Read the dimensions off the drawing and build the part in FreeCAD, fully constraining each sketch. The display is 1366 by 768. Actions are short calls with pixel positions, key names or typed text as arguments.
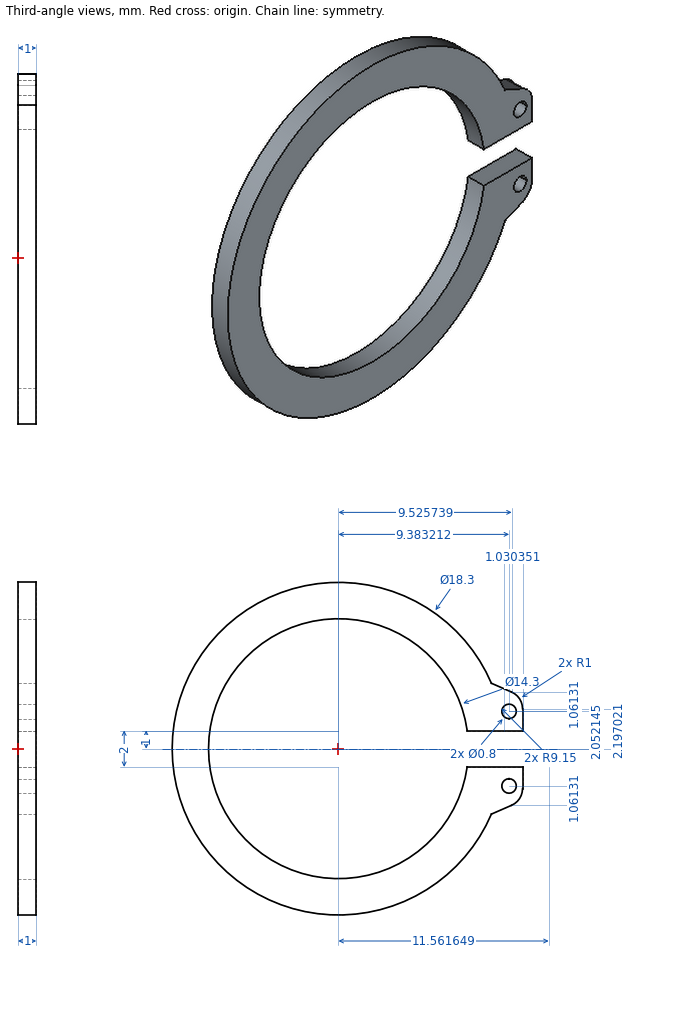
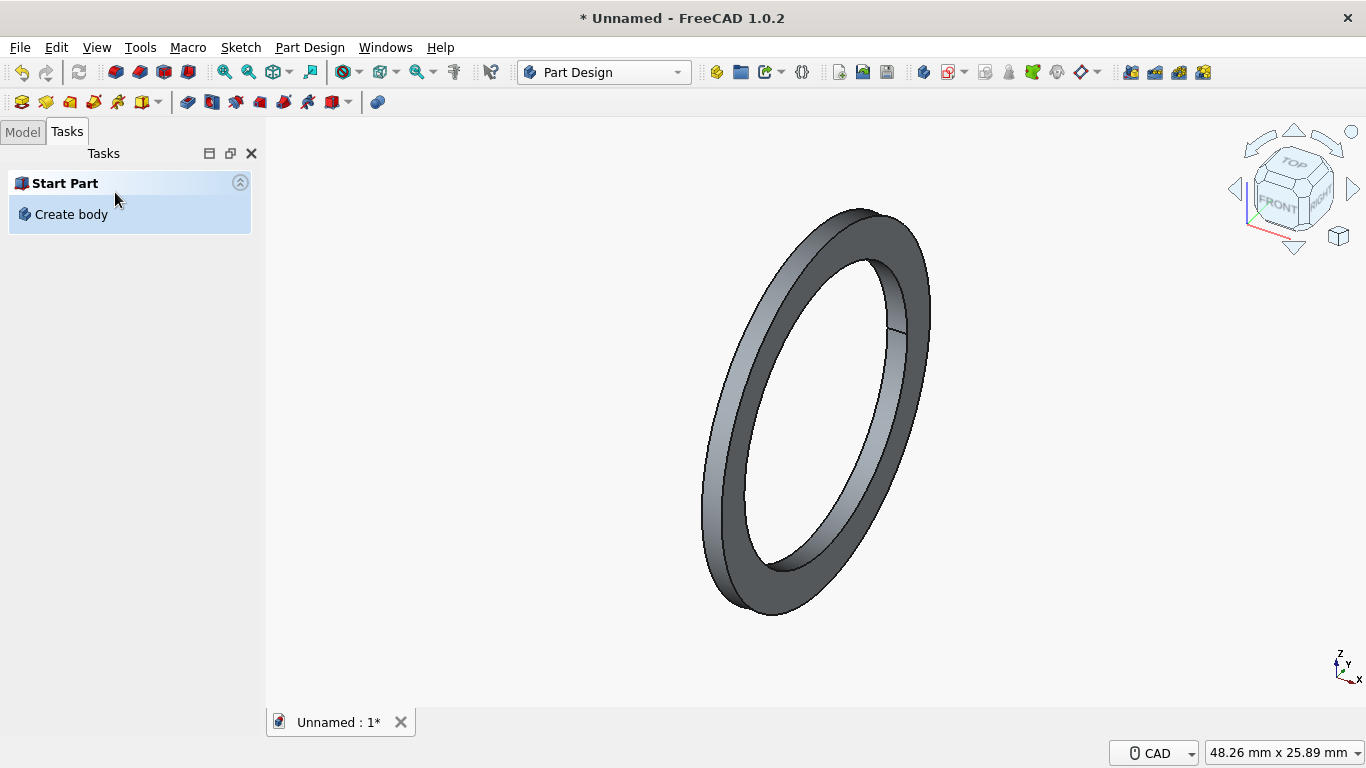
click(915, 374)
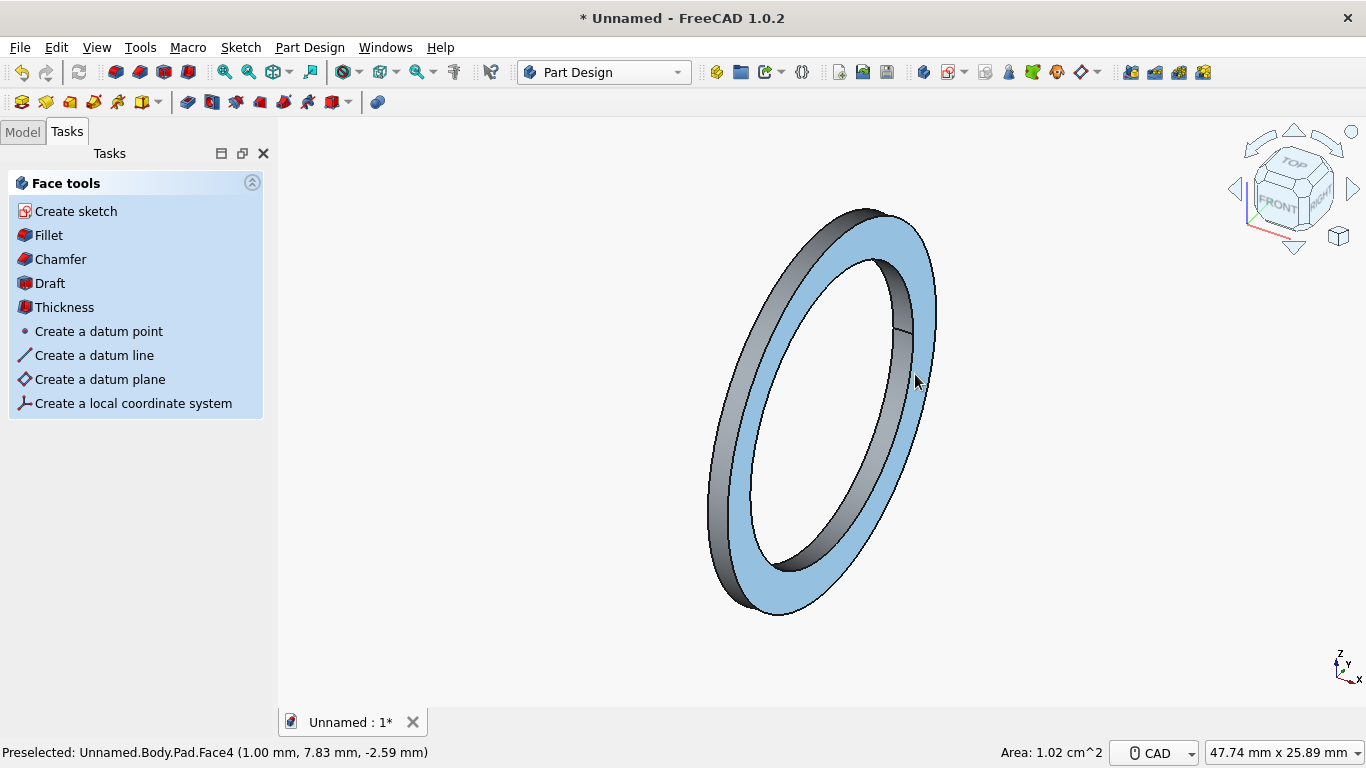
click(948, 72)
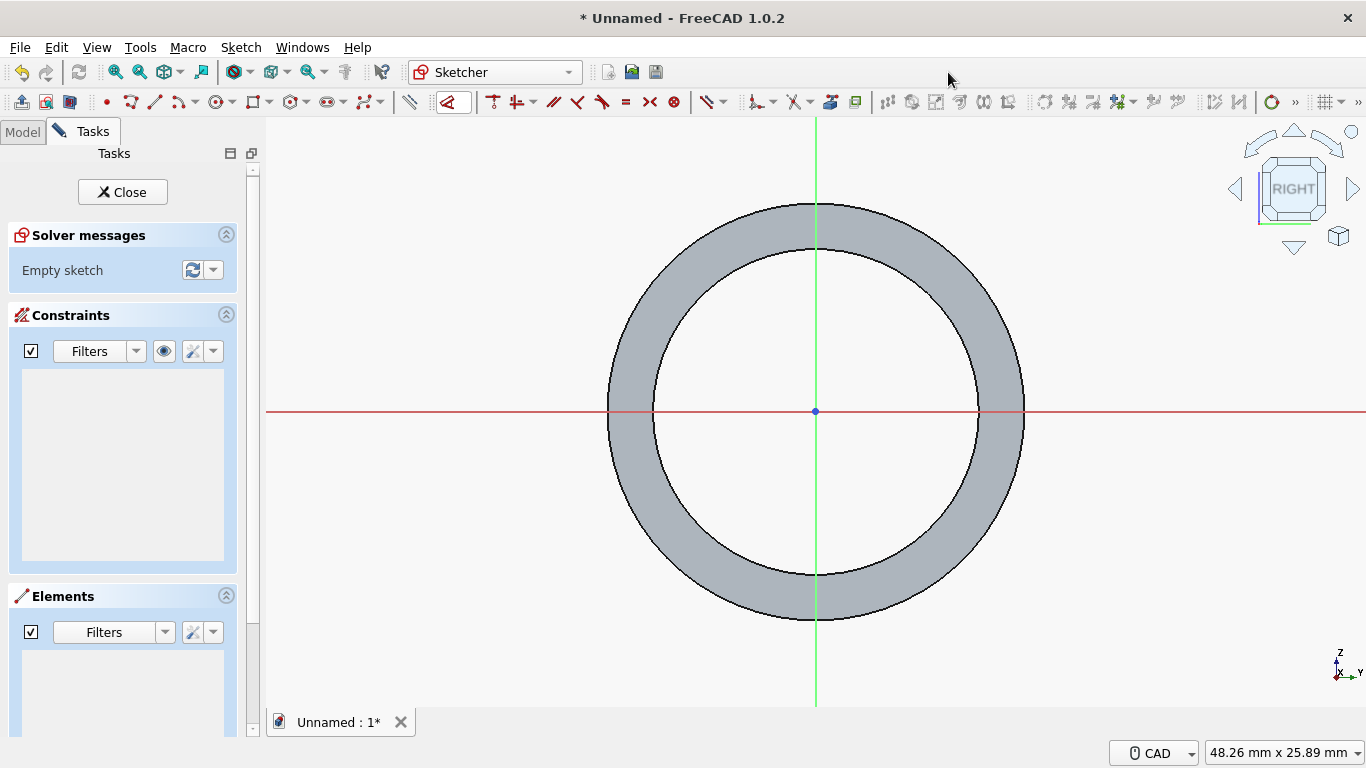
scroll(1111, 412, up, 4)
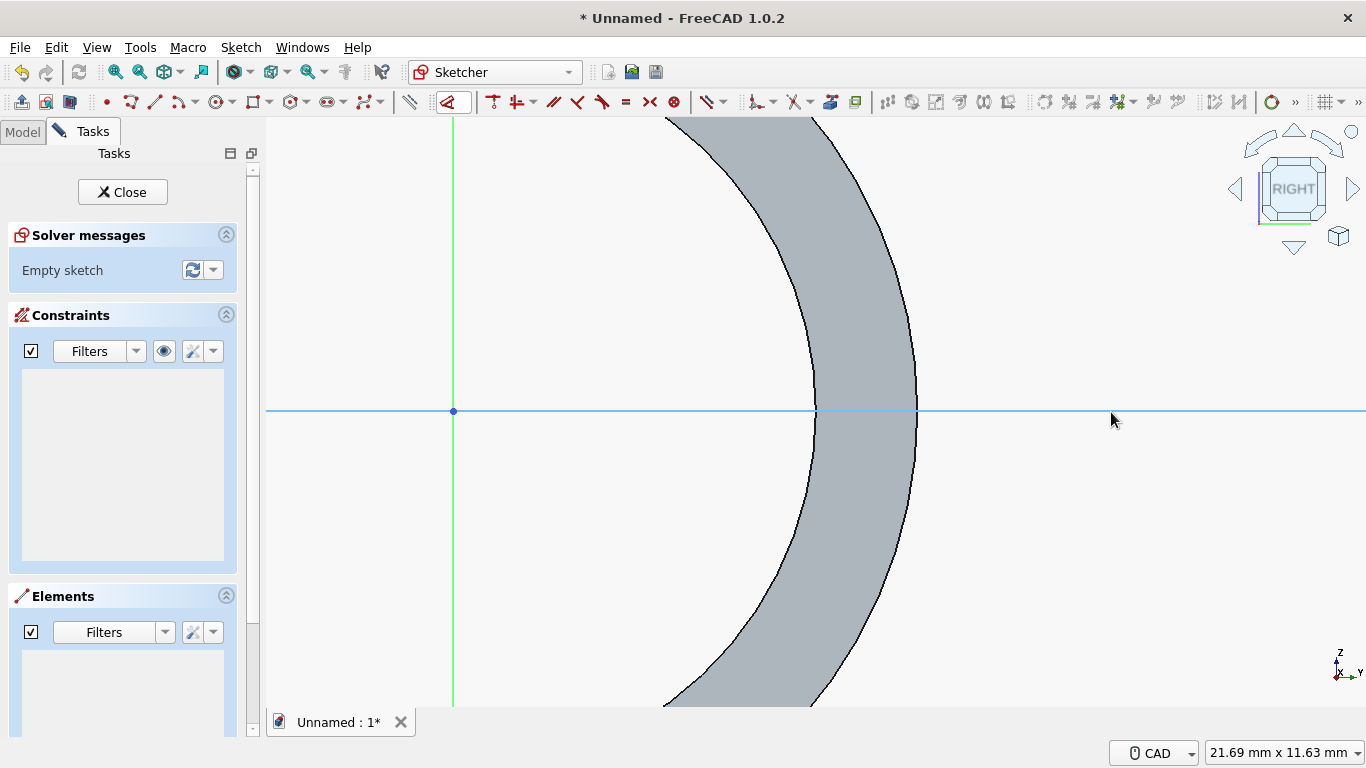
click(254, 102)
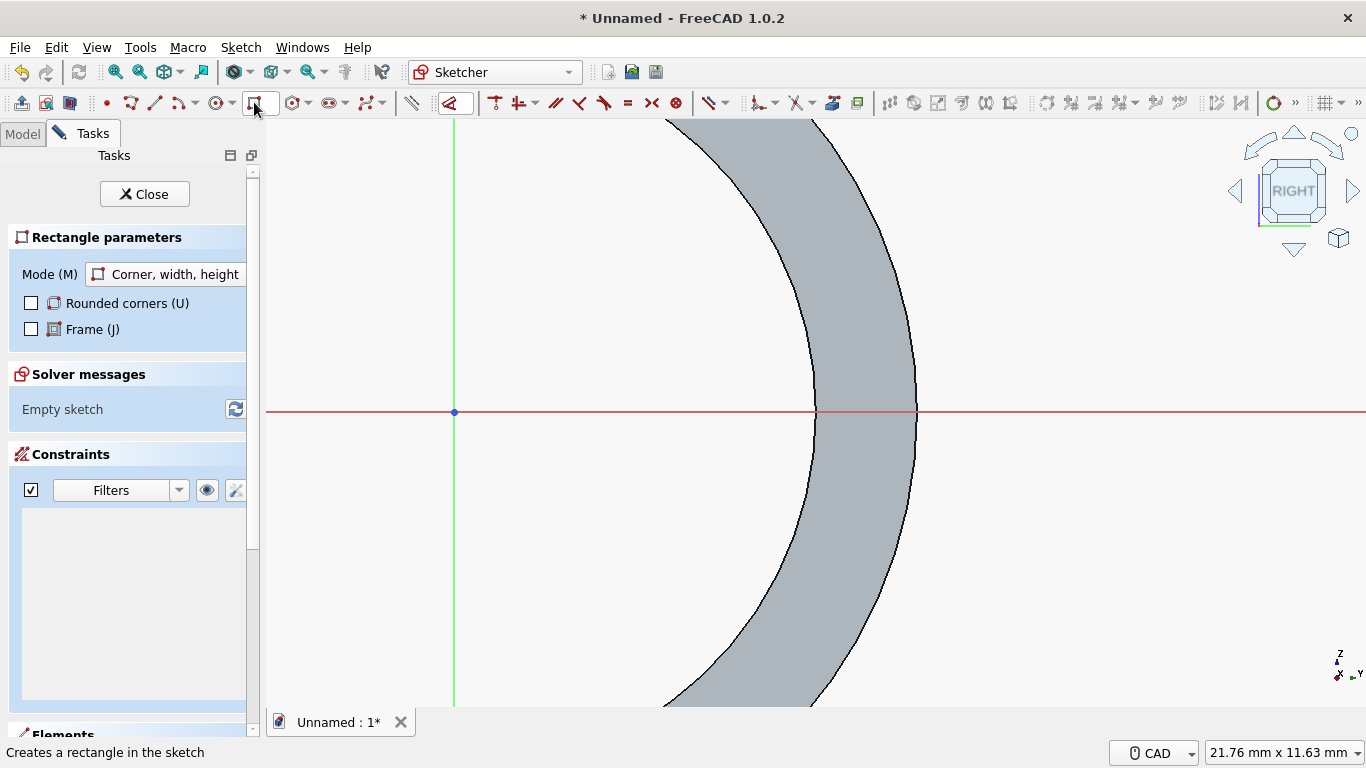
click(454, 362)
click(1039, 463)
key(Escape)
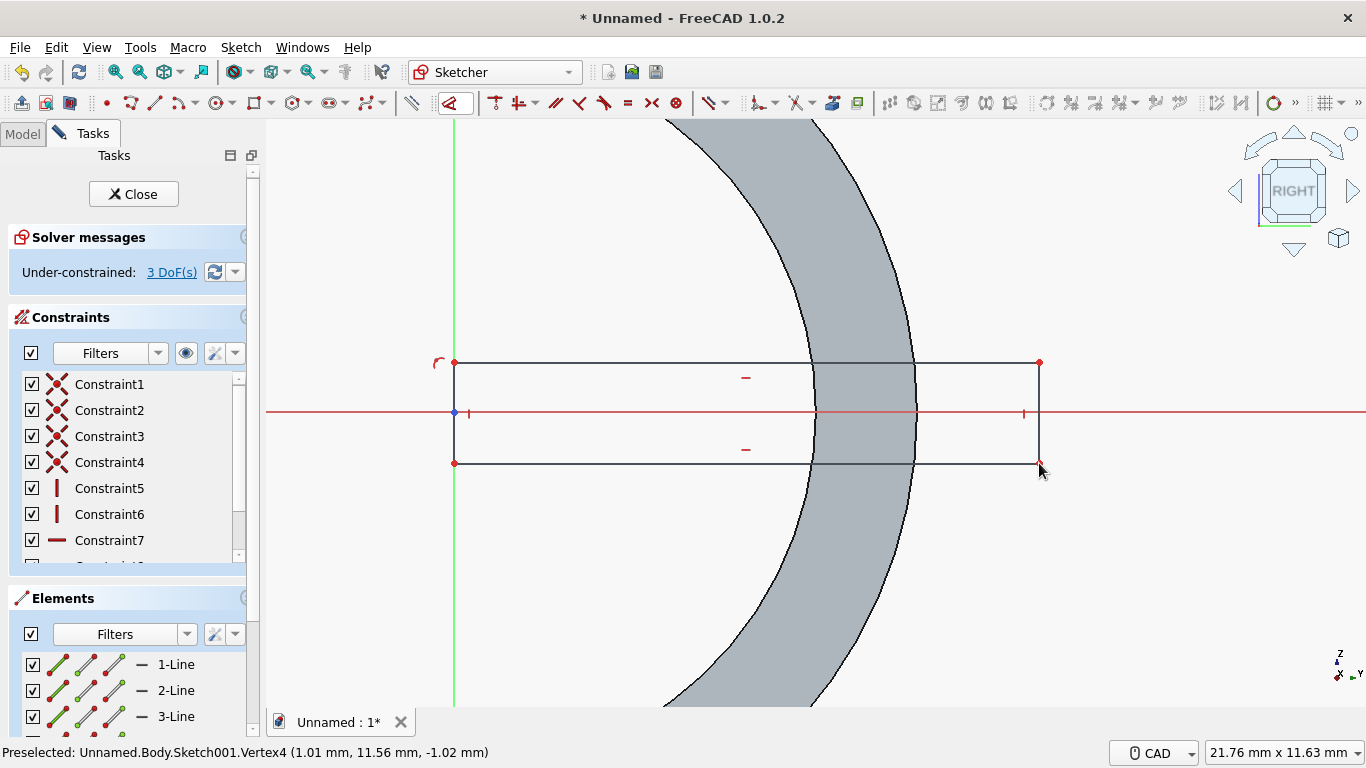
click(454, 393)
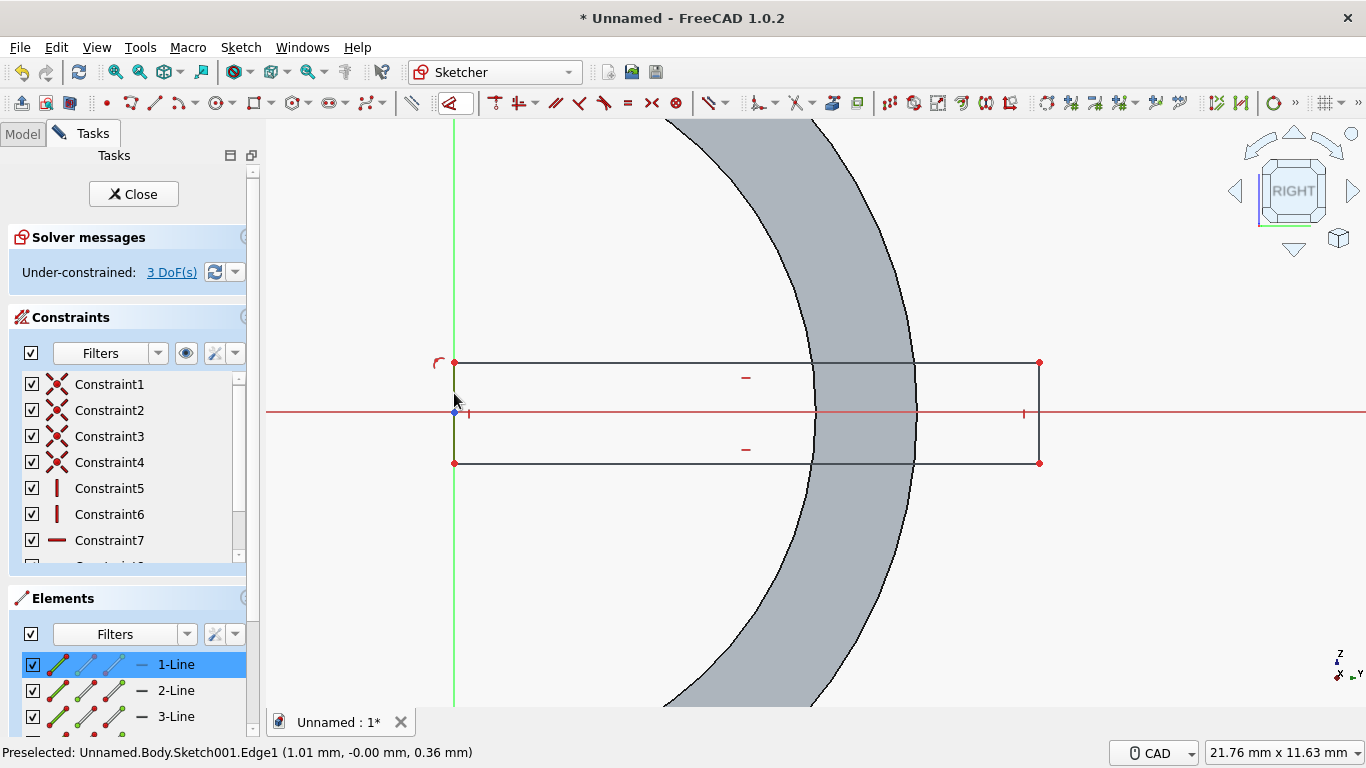
key(i)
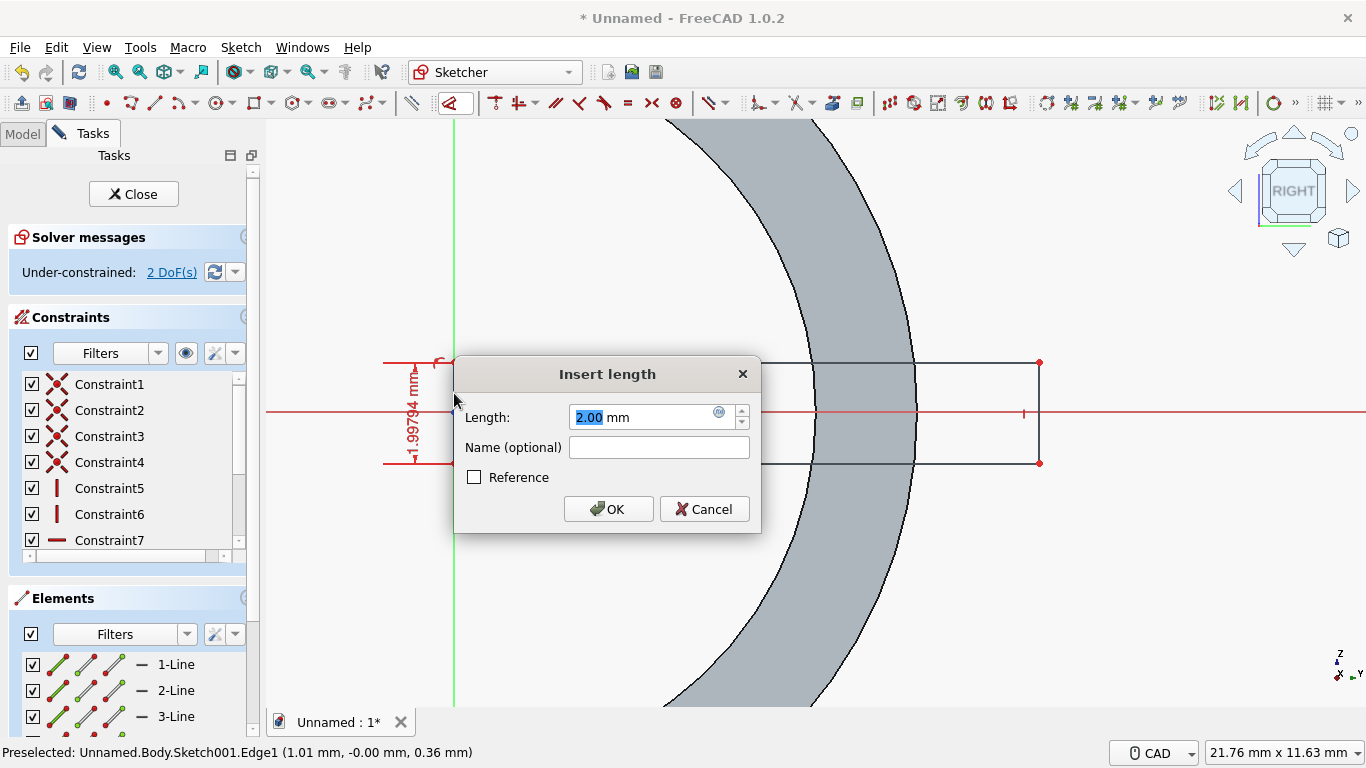
text(2)
key(Return)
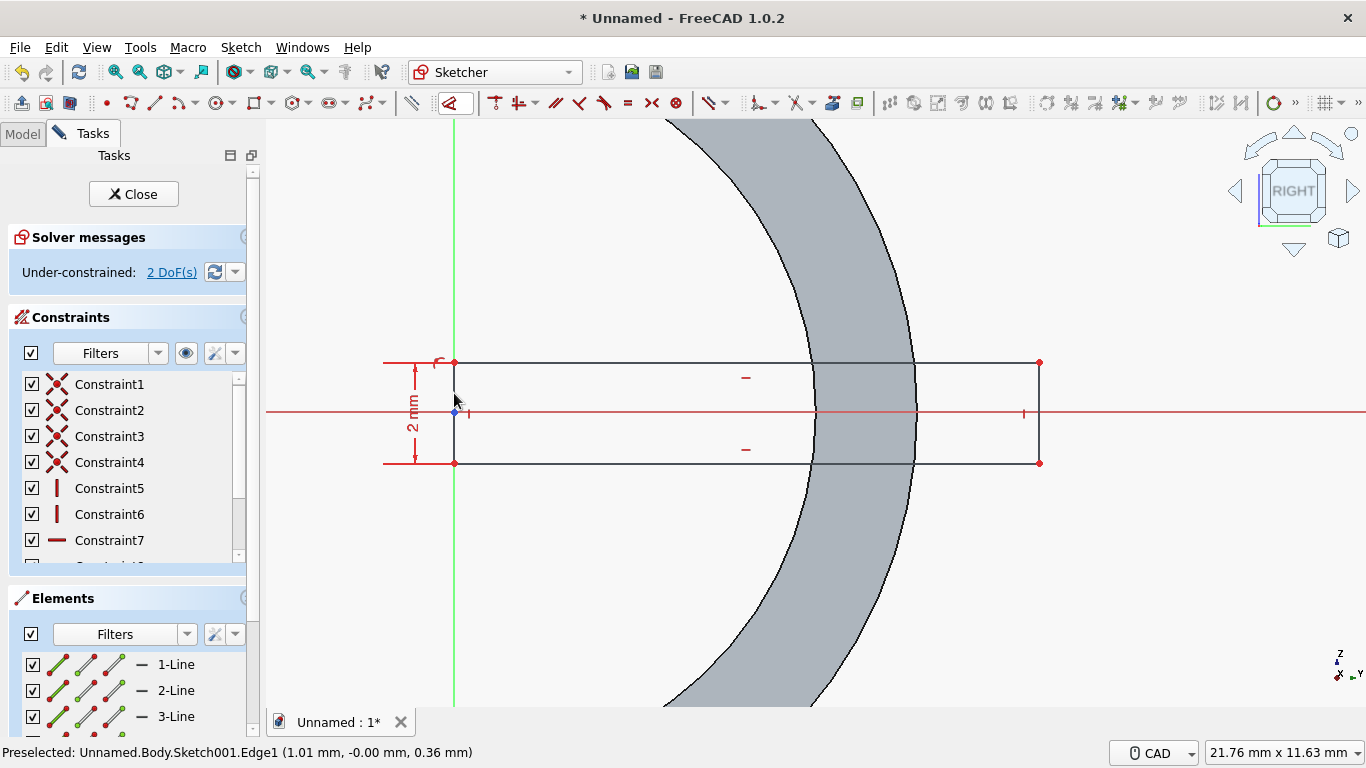
click(454, 363)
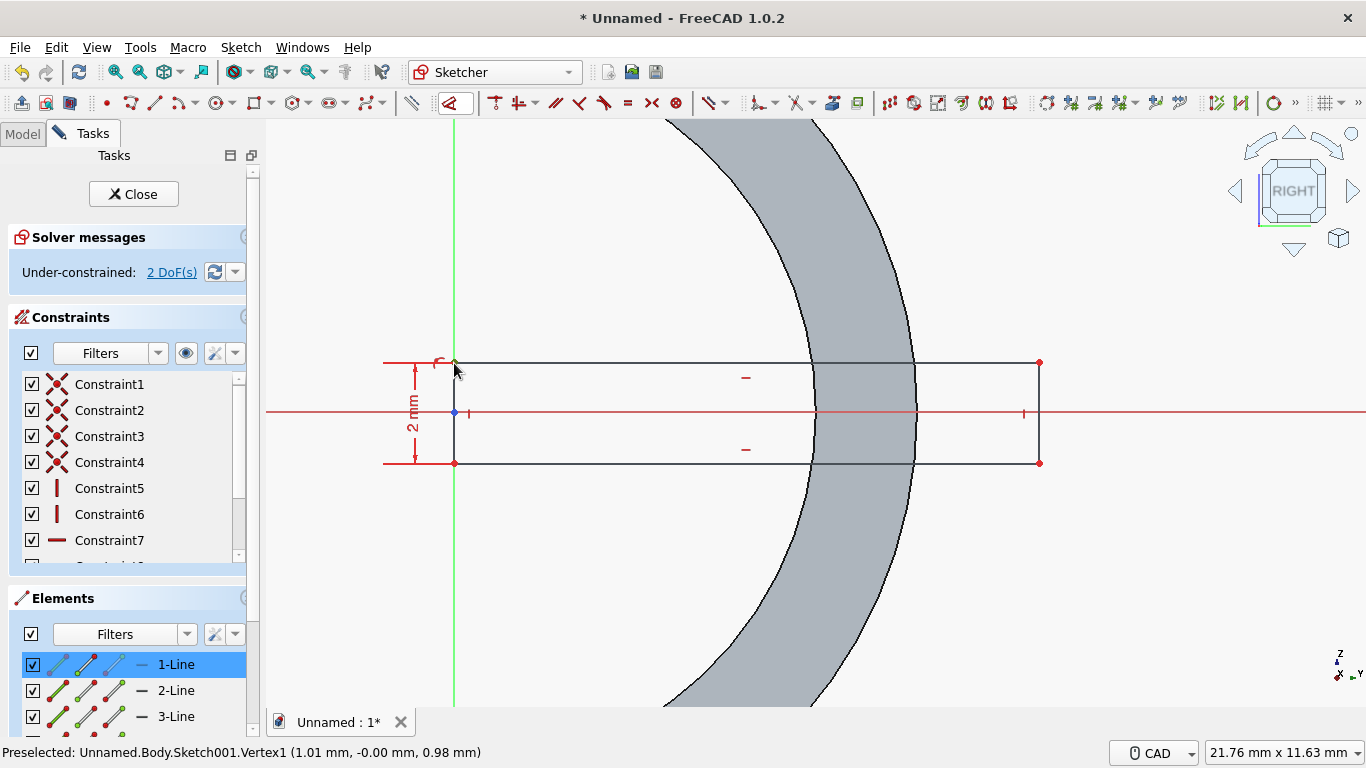
click(468, 104)